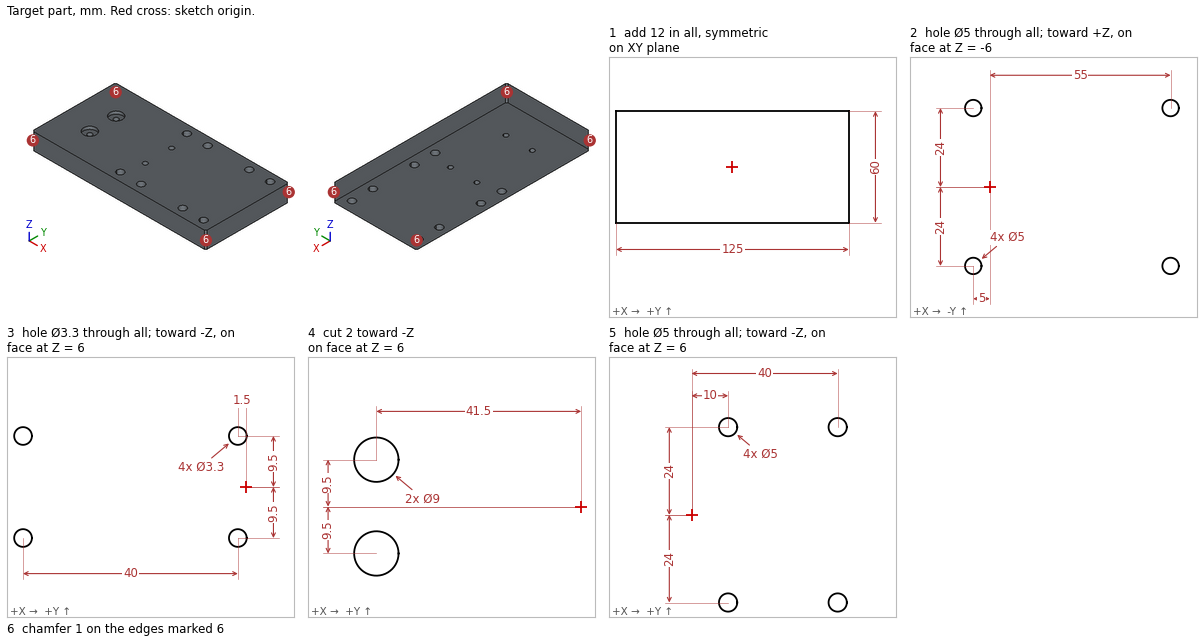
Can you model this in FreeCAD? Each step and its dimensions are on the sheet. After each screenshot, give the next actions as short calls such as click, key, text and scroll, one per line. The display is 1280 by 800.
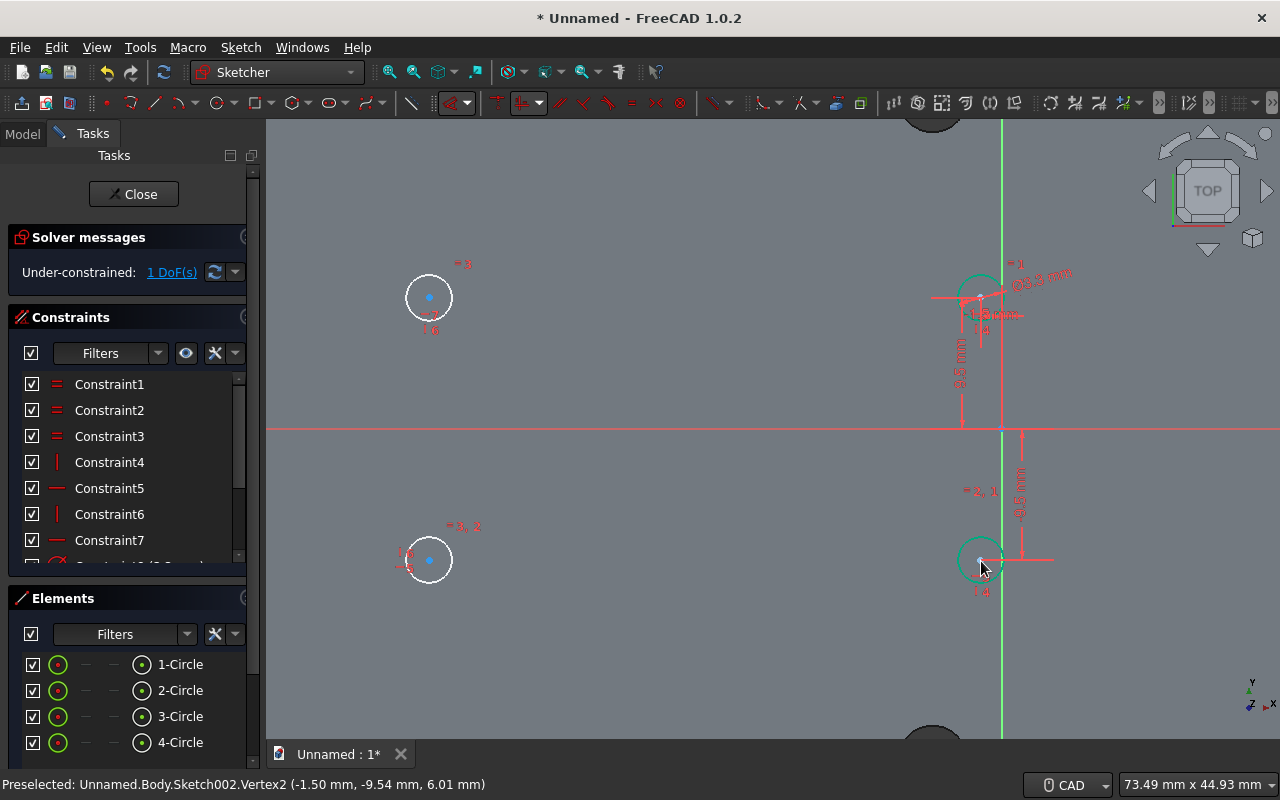
click(981, 560)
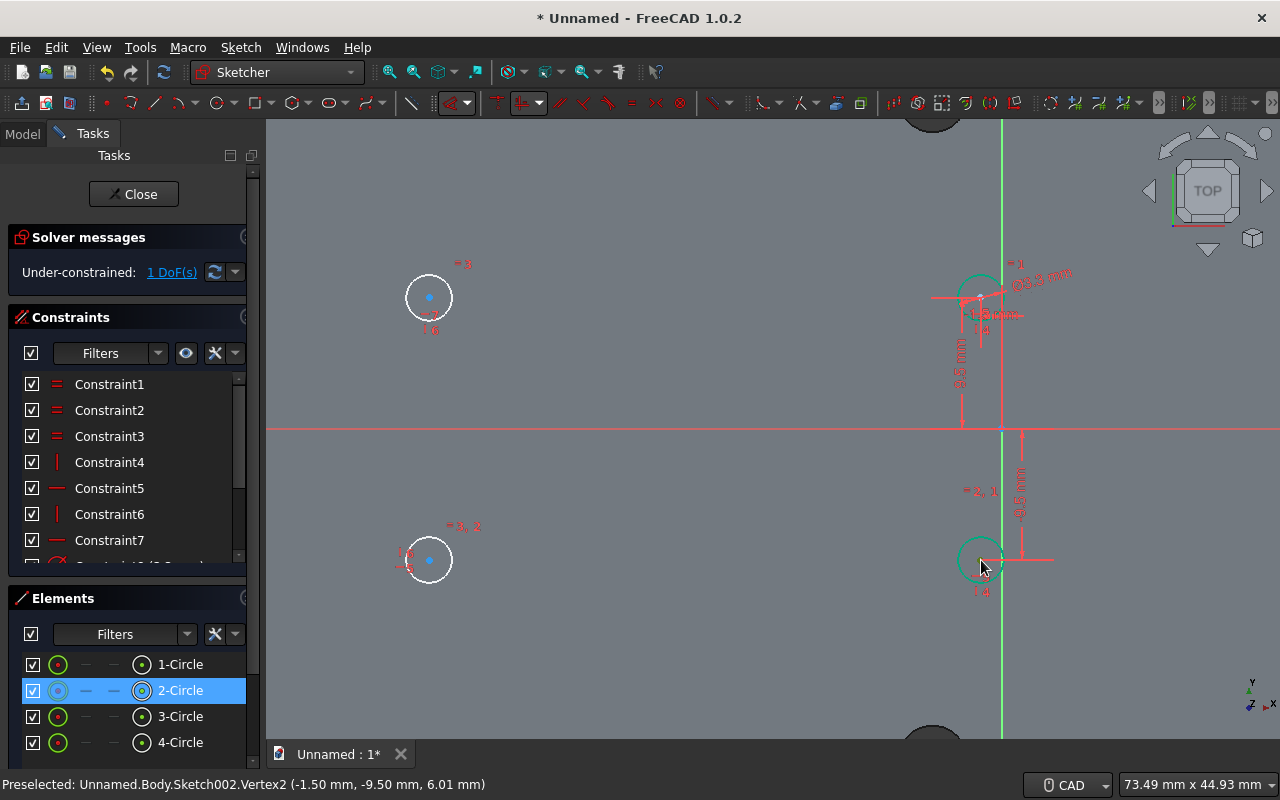
click(429, 560)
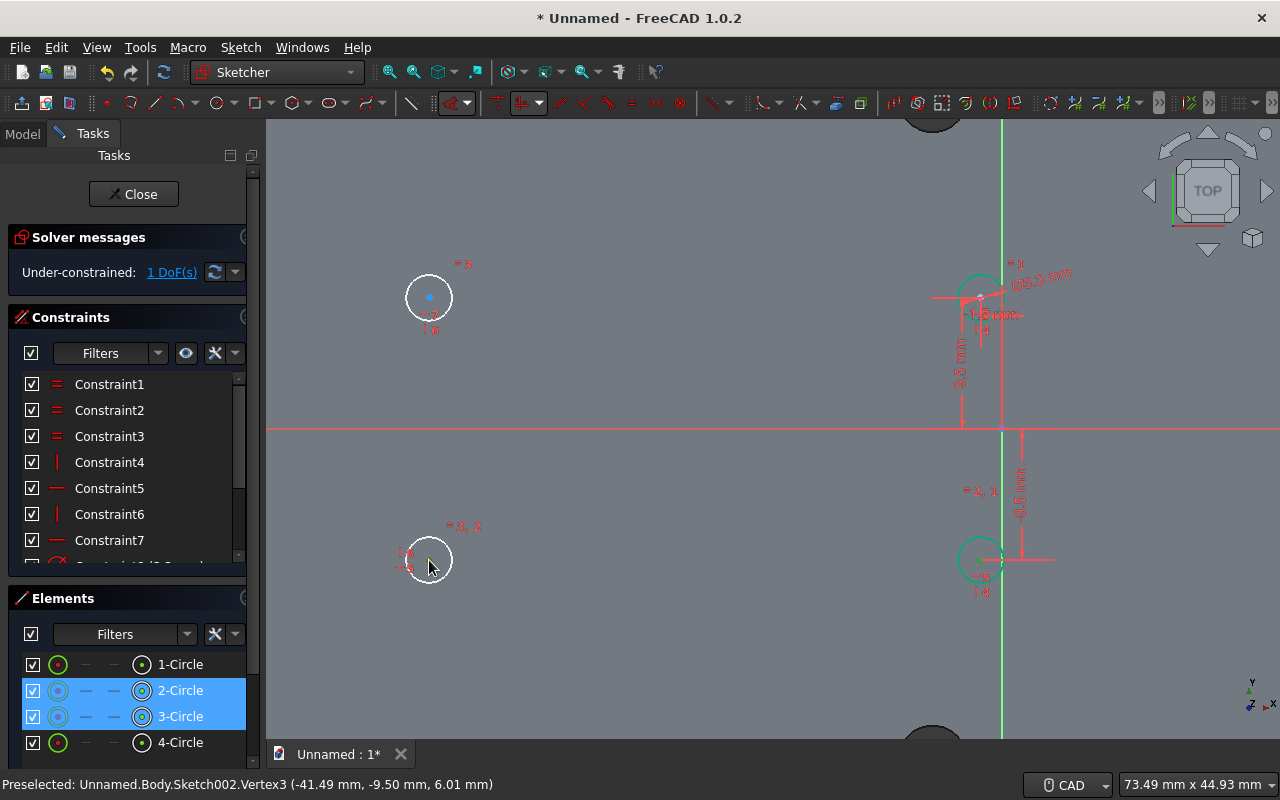
click(470, 104)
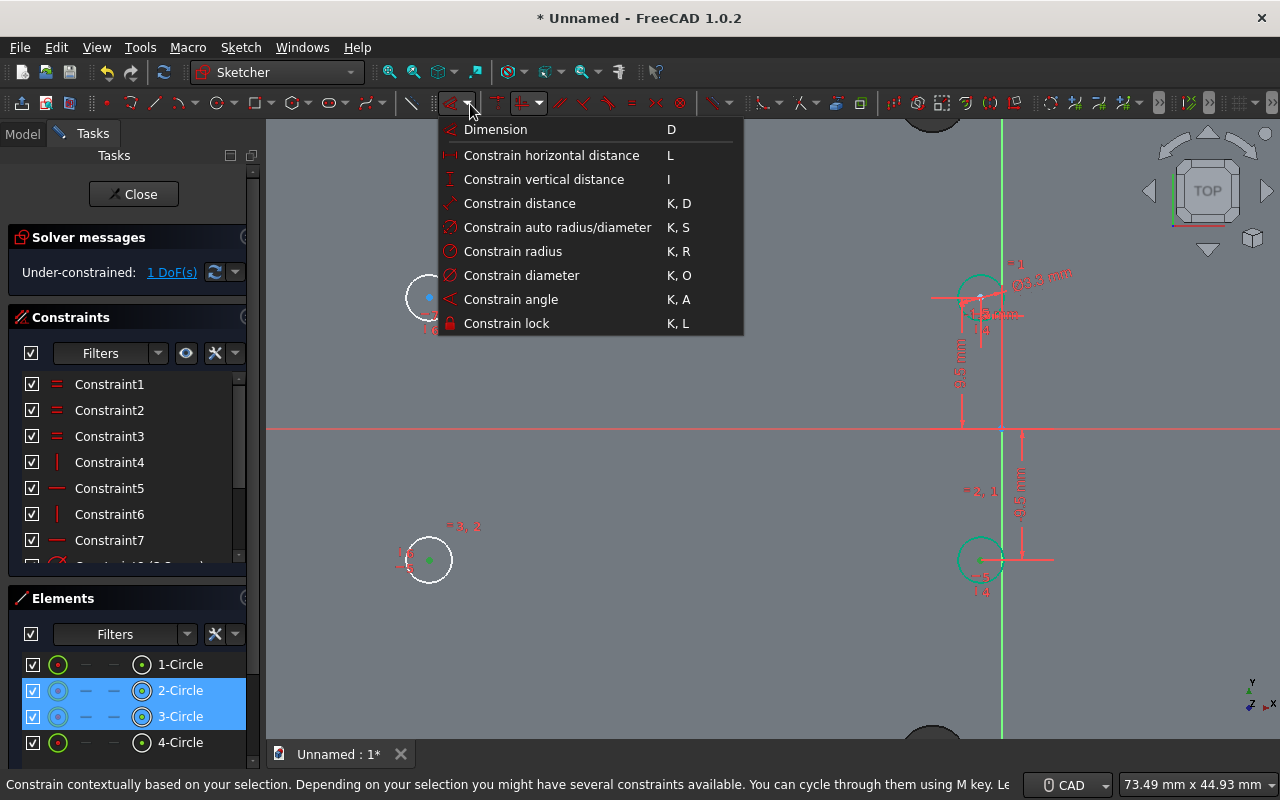
click(591, 155)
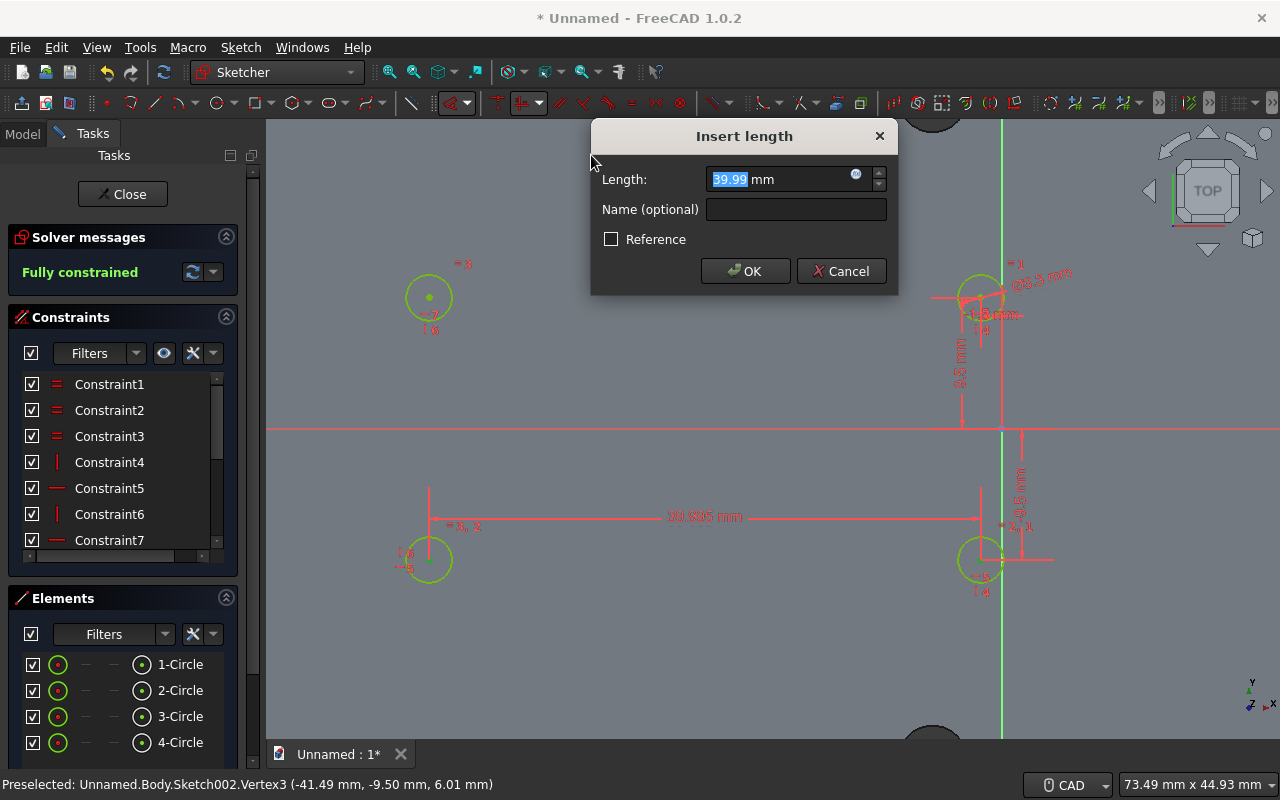
text(40)
key(Return)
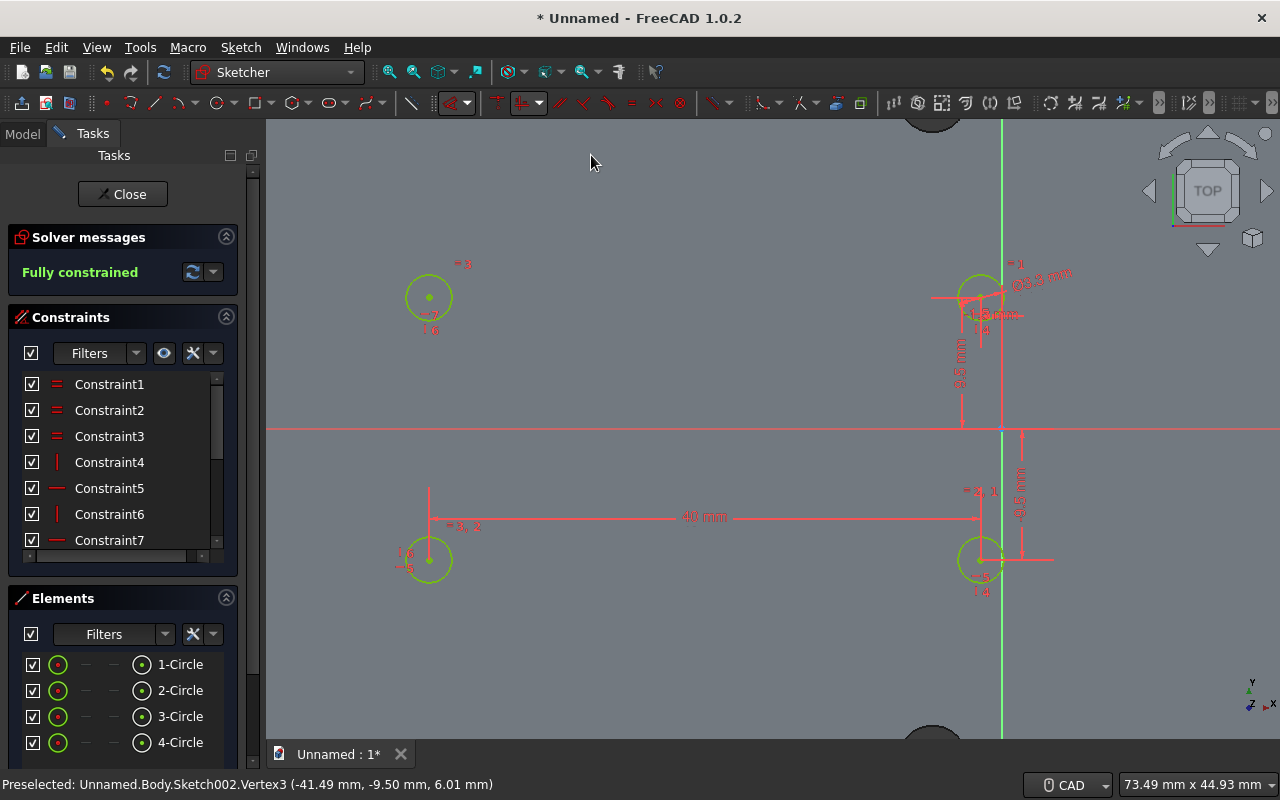
click(123, 194)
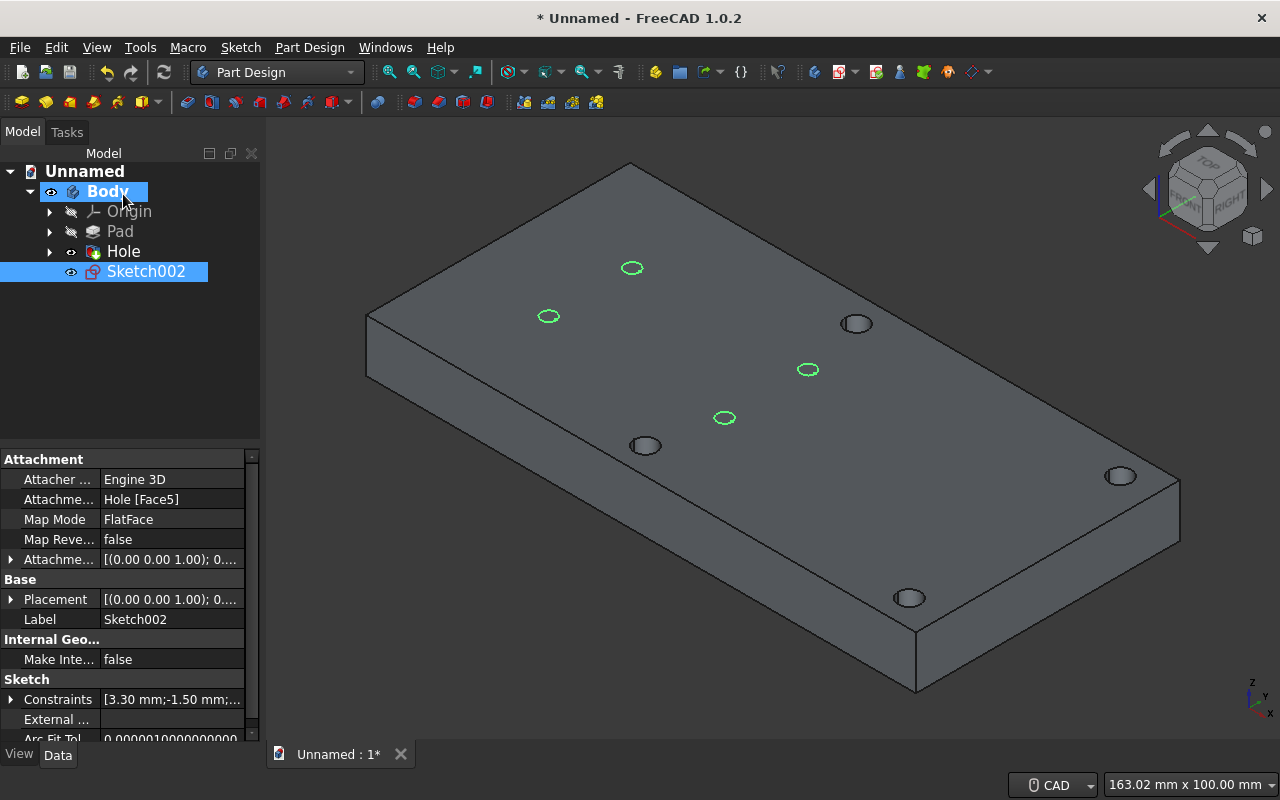
click(212, 102)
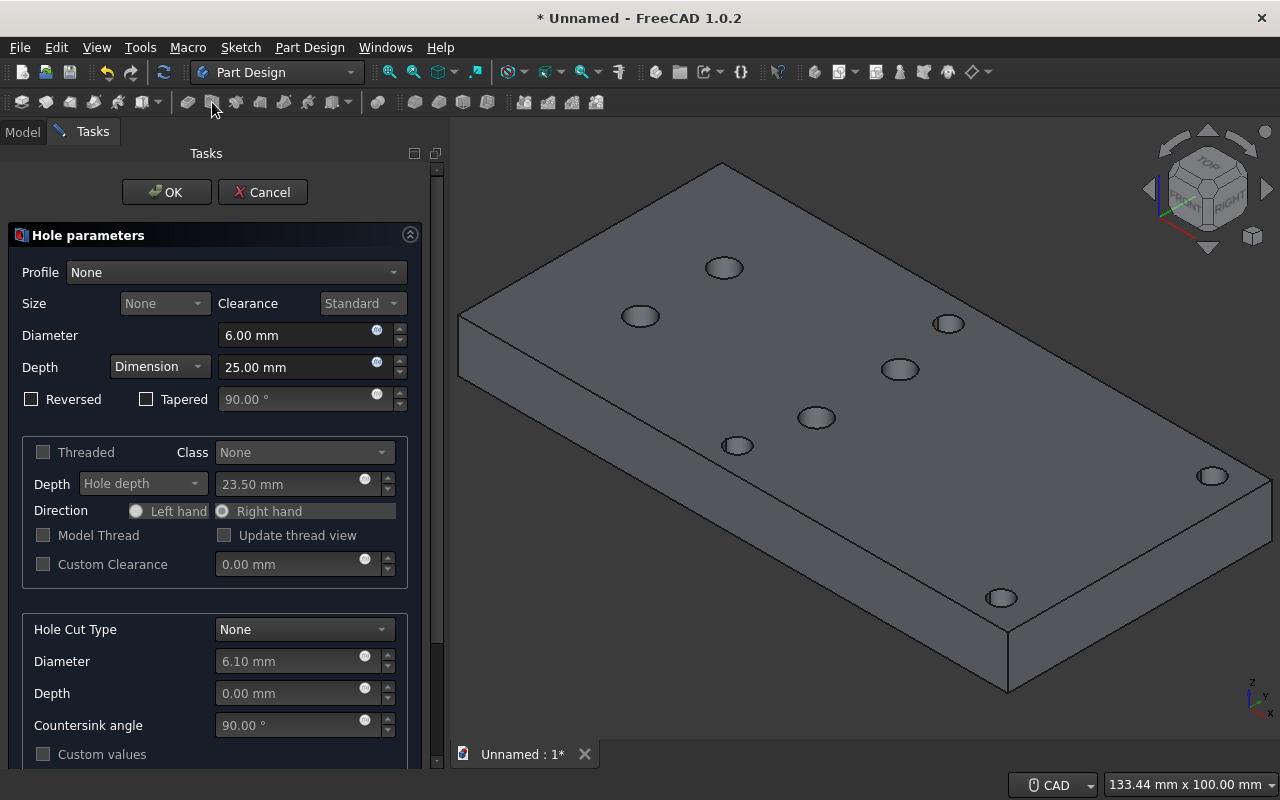
triple_click(305, 335)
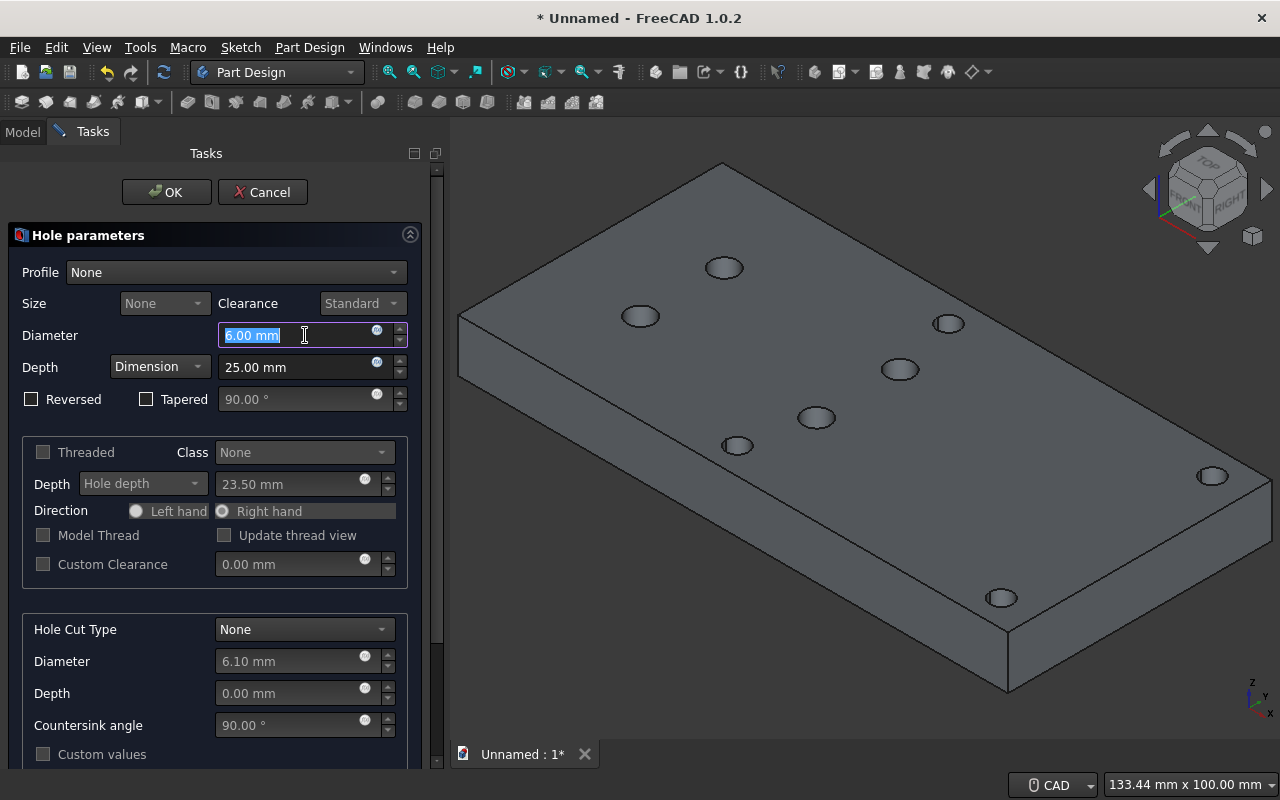
text(3.3)
key(Tab)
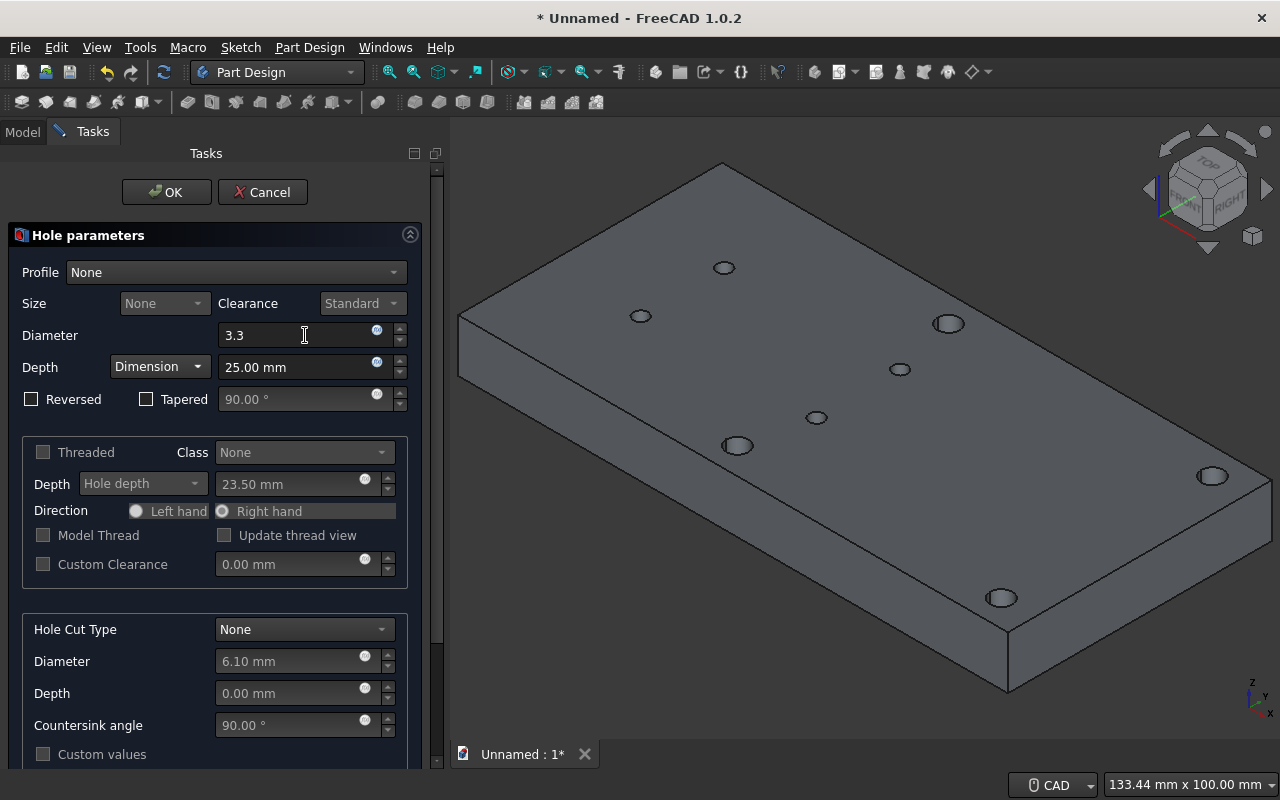
click(161, 366)